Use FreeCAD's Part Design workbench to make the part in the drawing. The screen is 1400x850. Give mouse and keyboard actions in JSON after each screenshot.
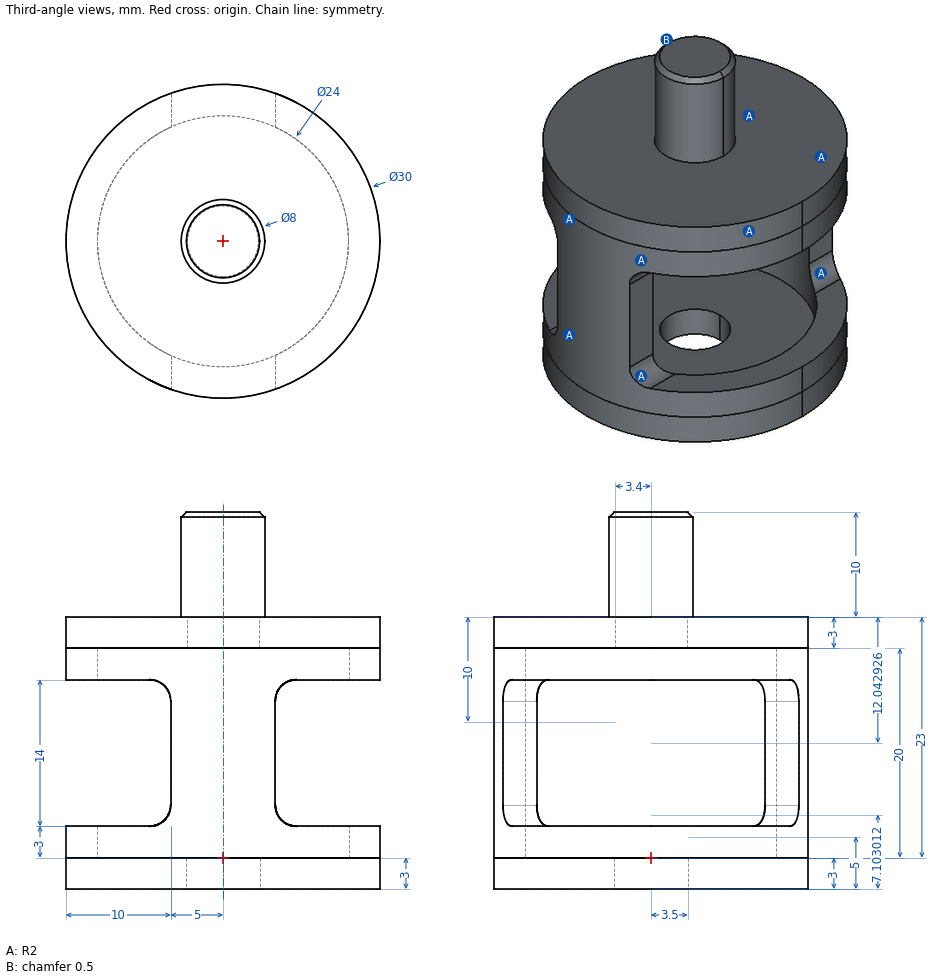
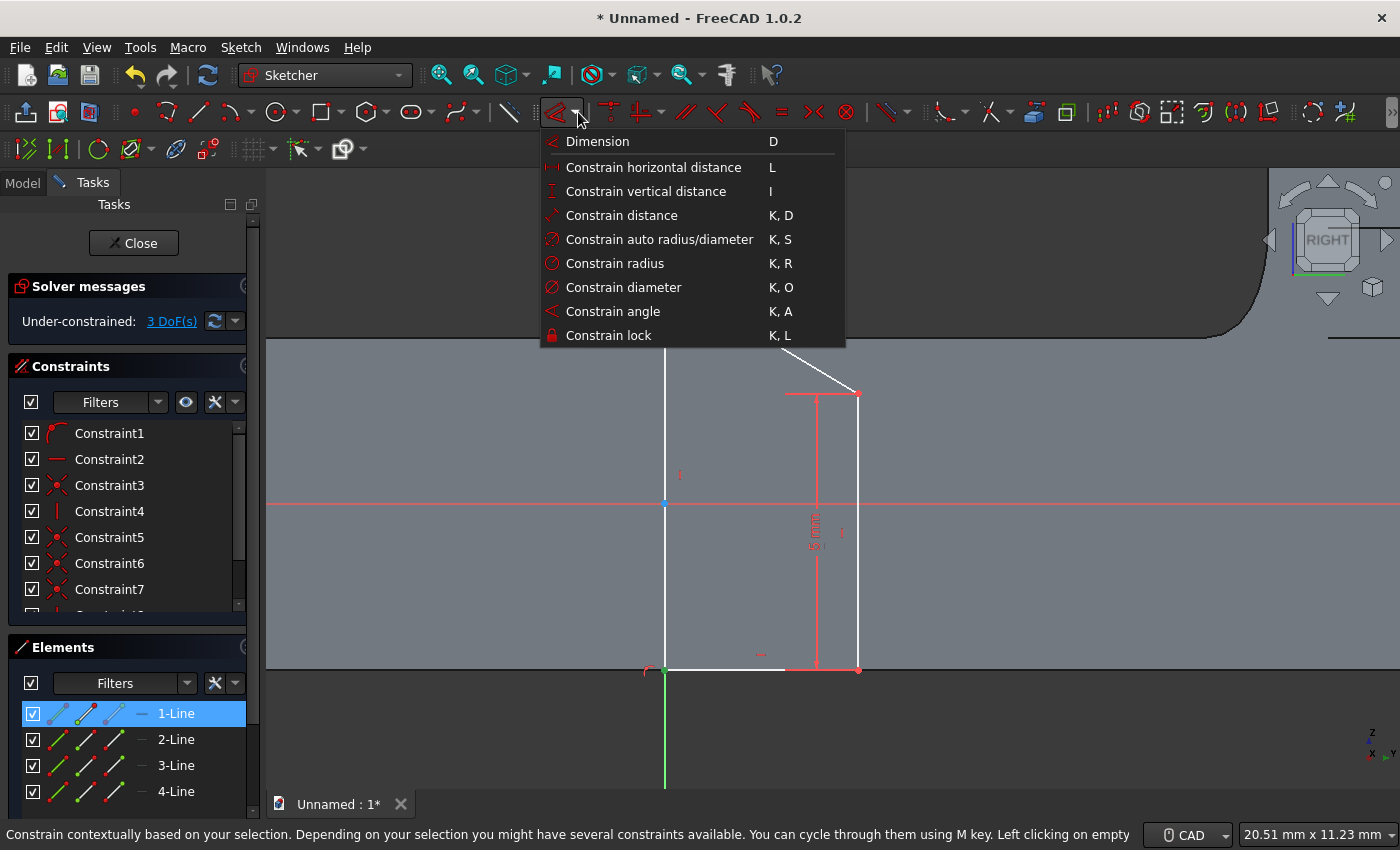
{"action": "left_click", "coordinate": [693, 191]}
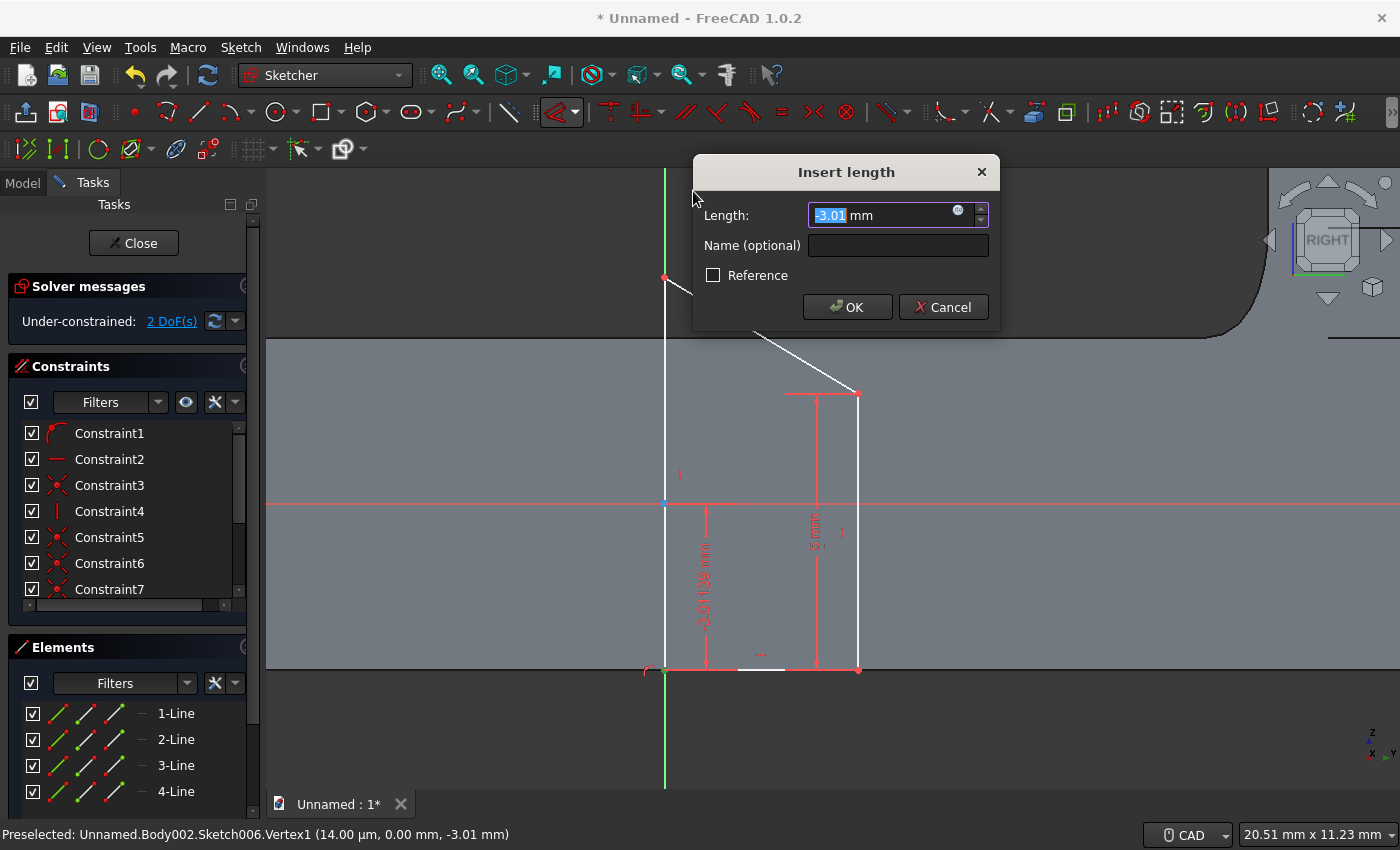
{"action": "type", "text": "-3"}
{"action": "key", "text": "Return"}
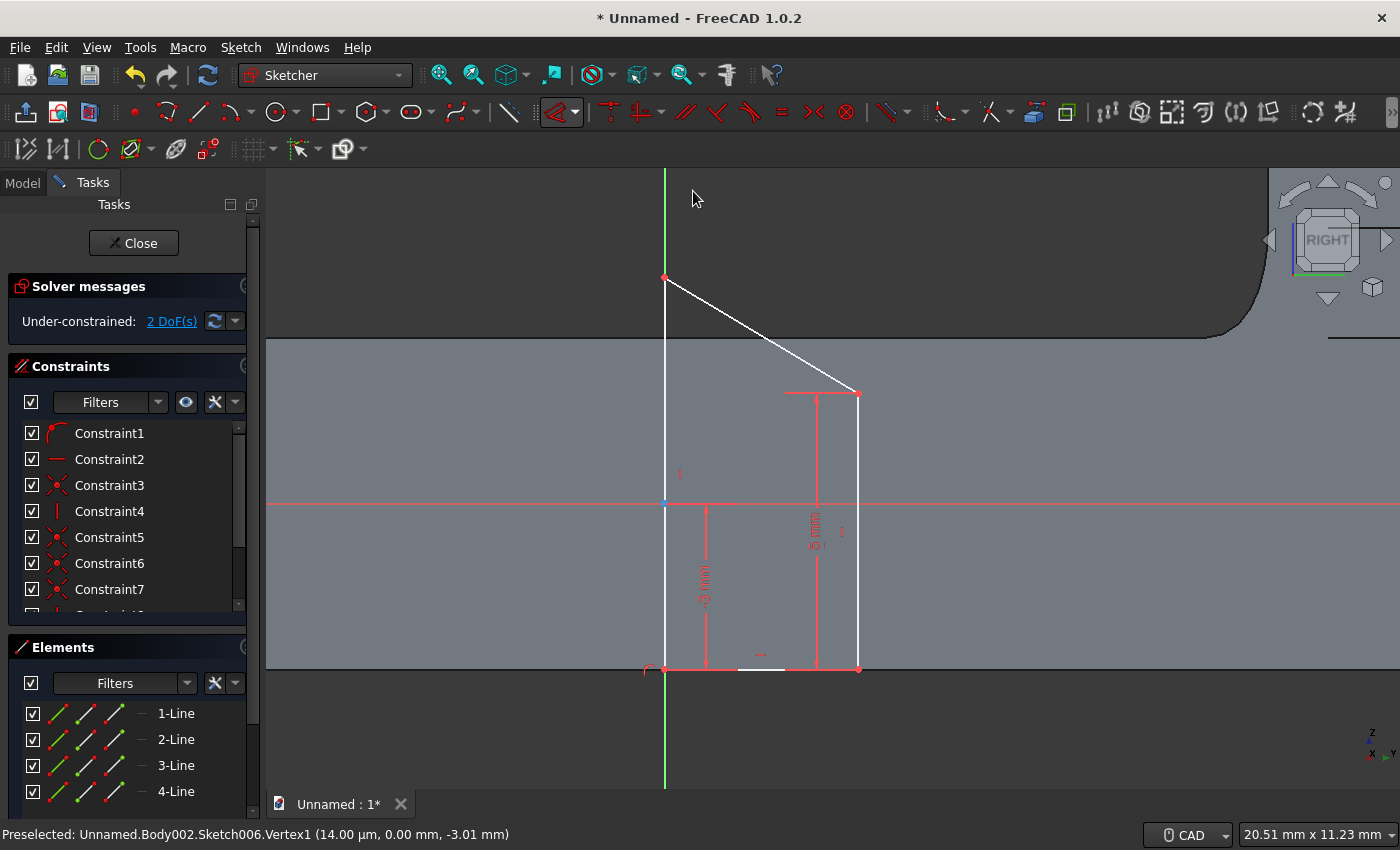
{"action": "left_click", "coordinate": [723, 670]}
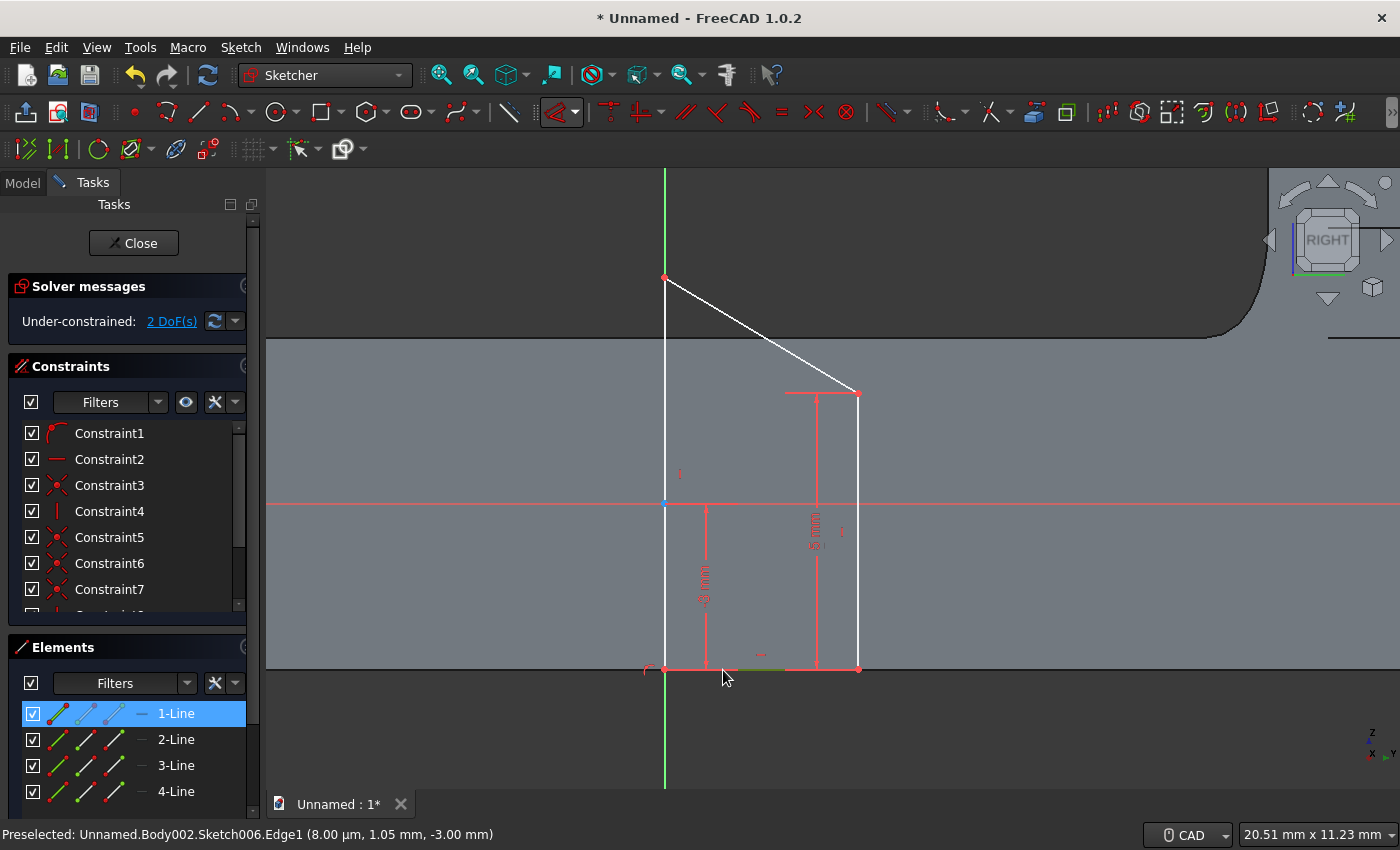
{"action": "key", "text": "l"}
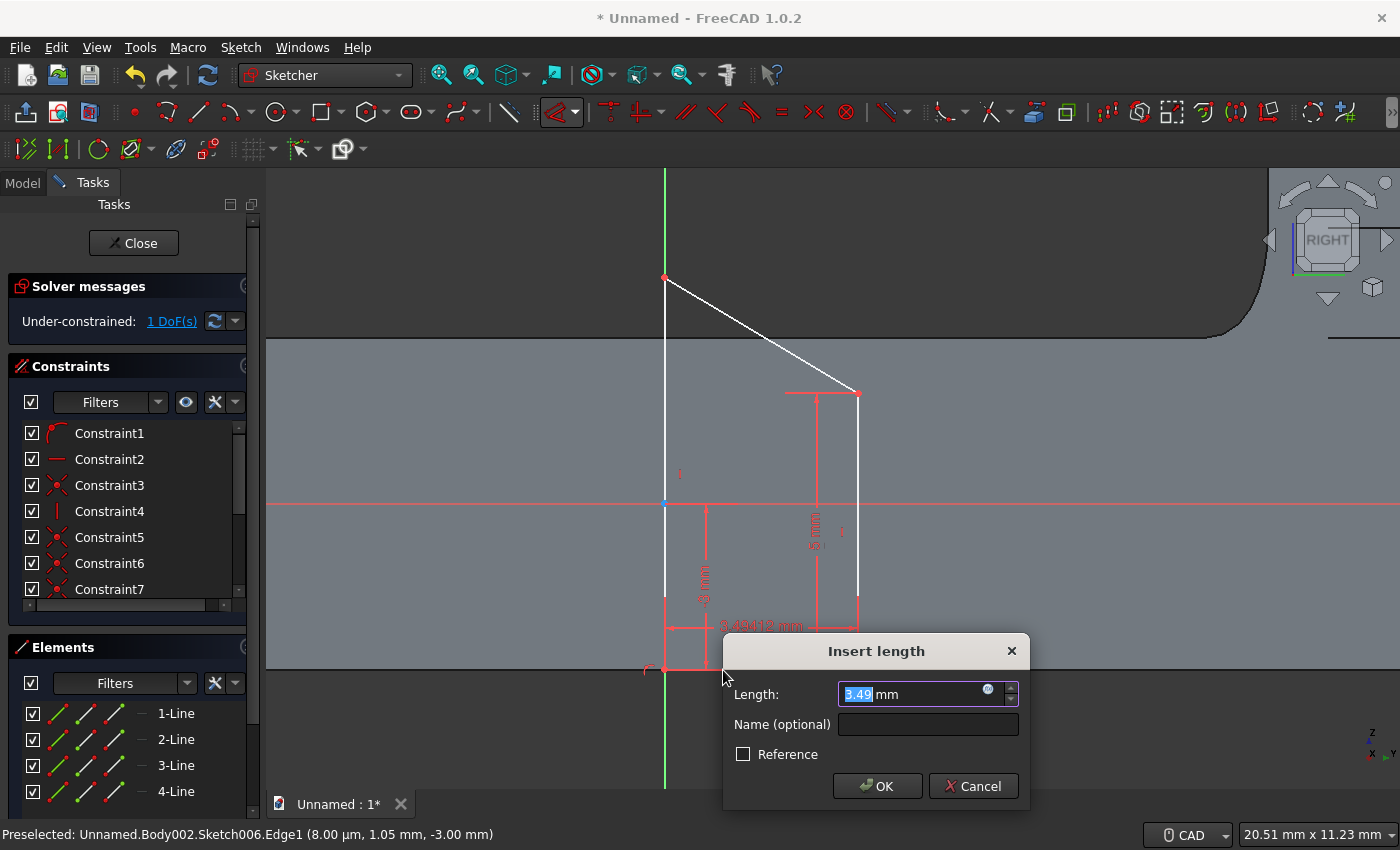
{"action": "type", "text": "3.5"}
{"action": "key", "text": "Return"}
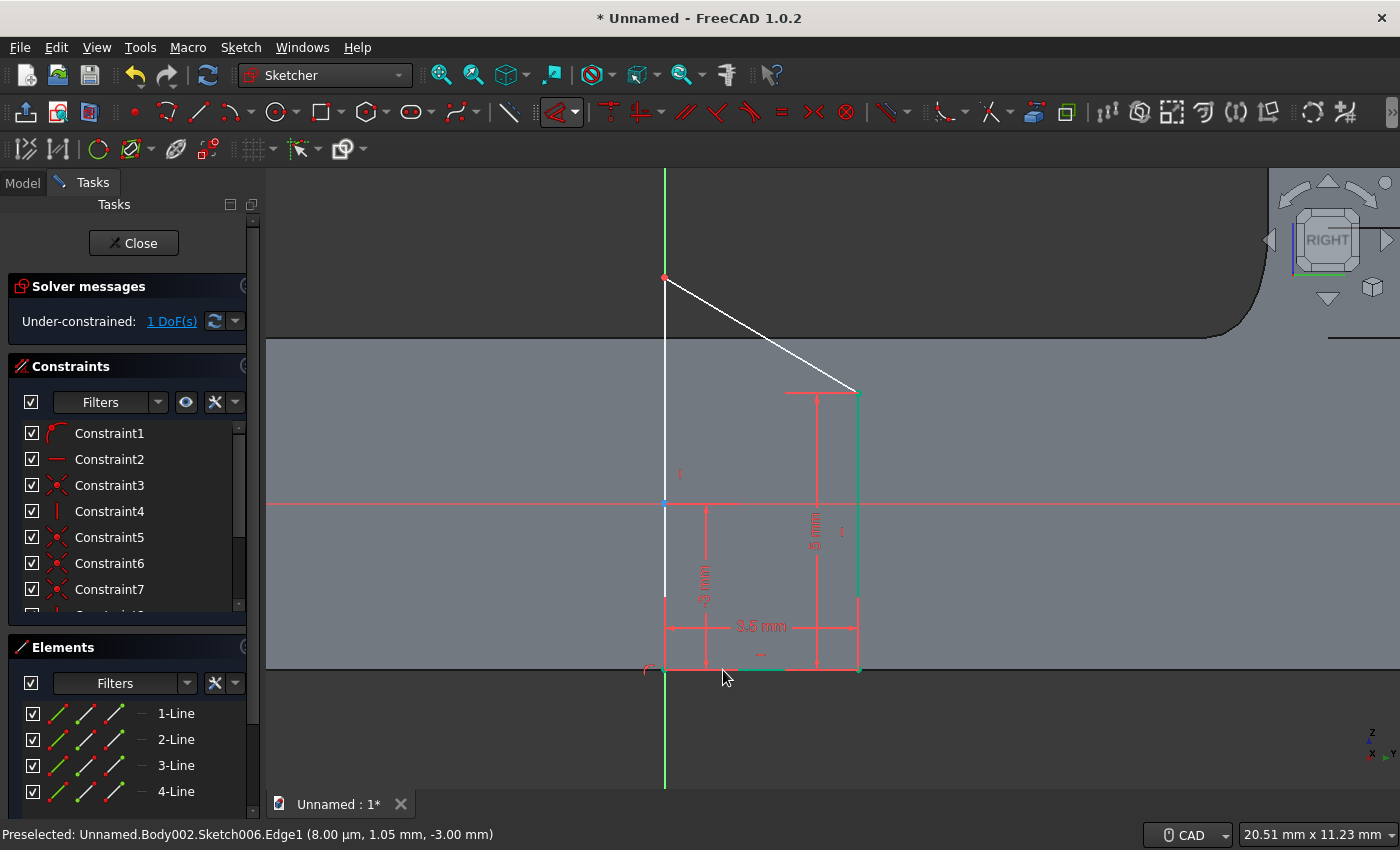
{"action": "left_click", "coordinate": [665, 396]}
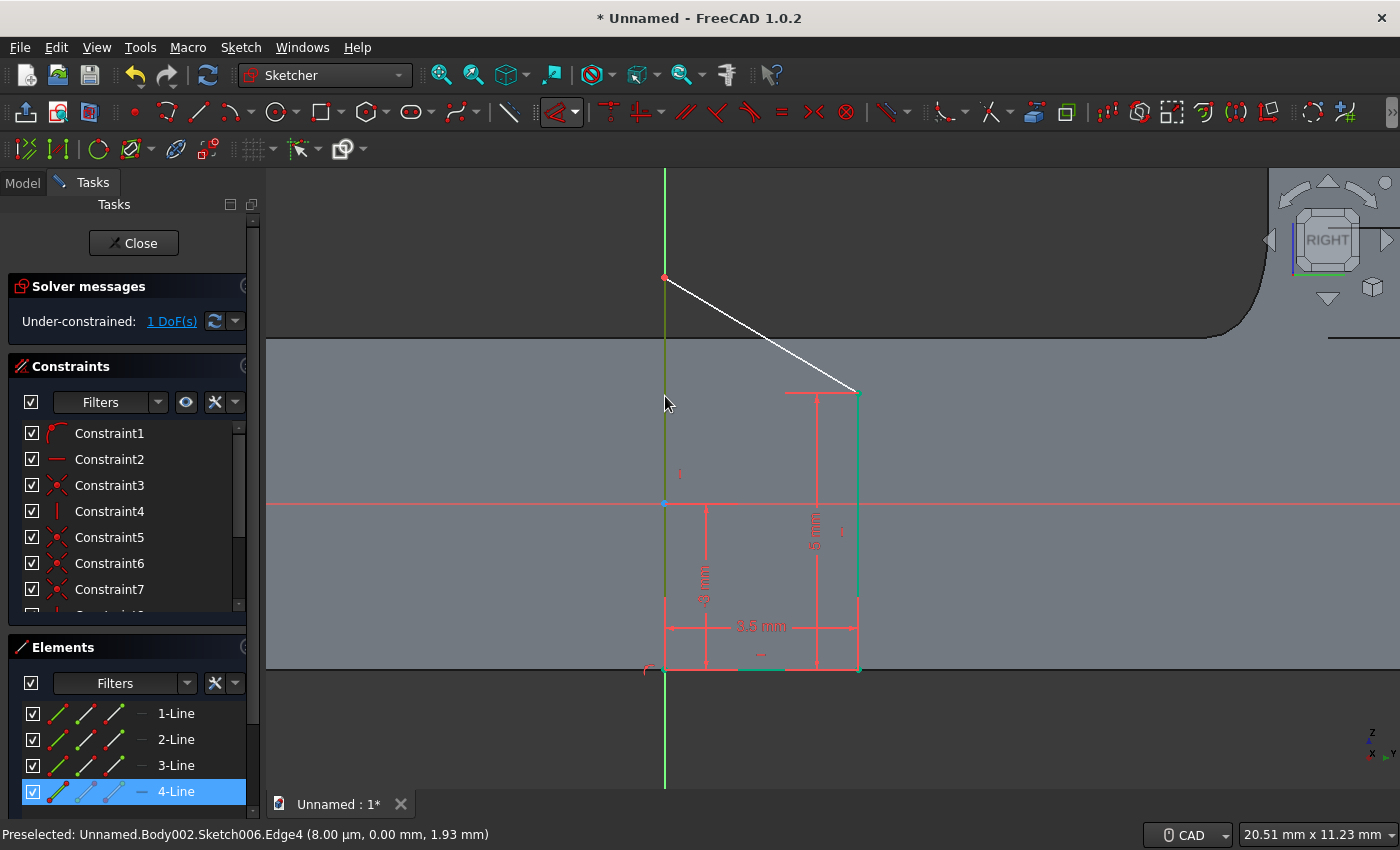
{"action": "key", "text": "i"}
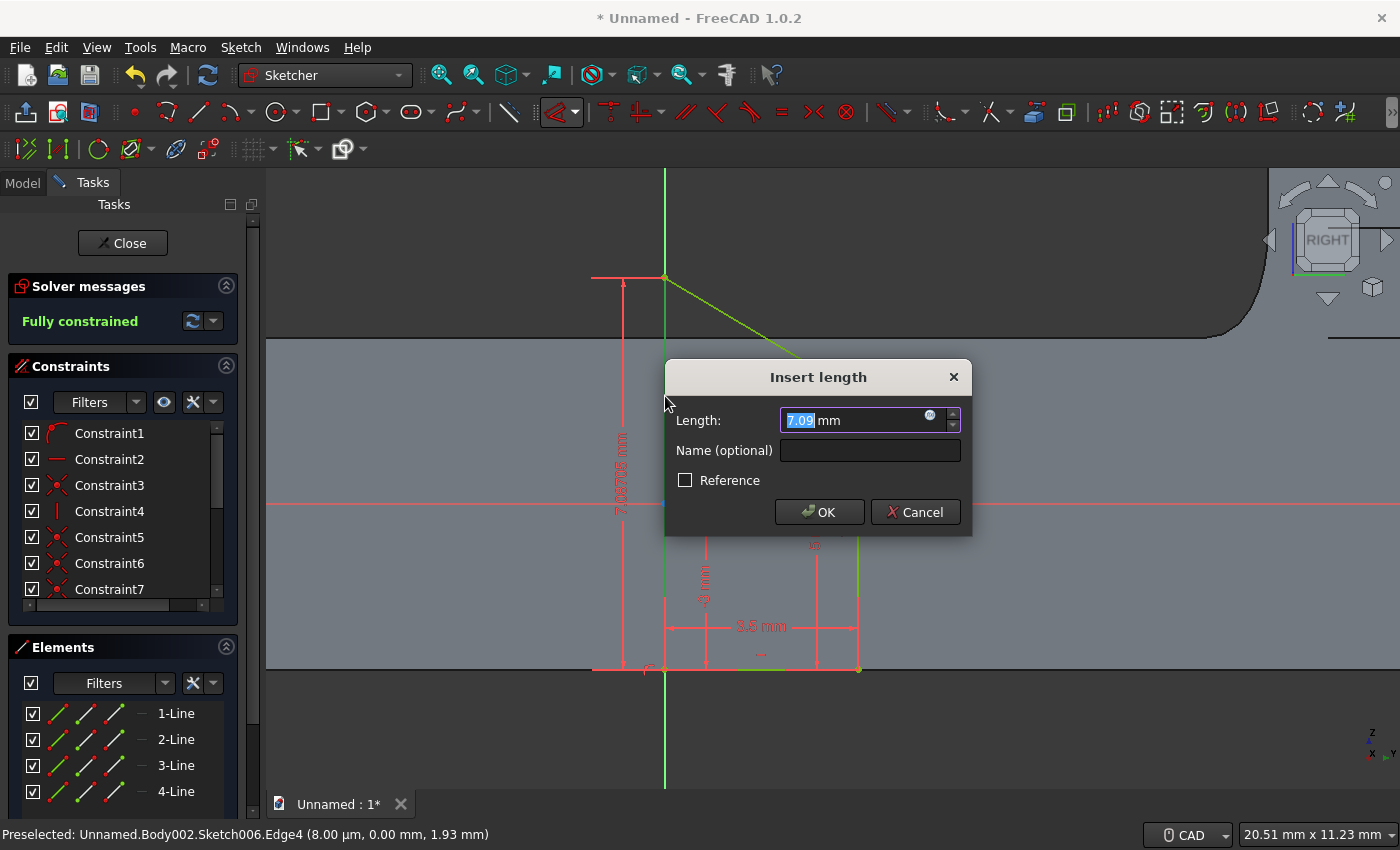
{"action": "type", "text": "7.103012"}
{"action": "key", "text": "Return"}